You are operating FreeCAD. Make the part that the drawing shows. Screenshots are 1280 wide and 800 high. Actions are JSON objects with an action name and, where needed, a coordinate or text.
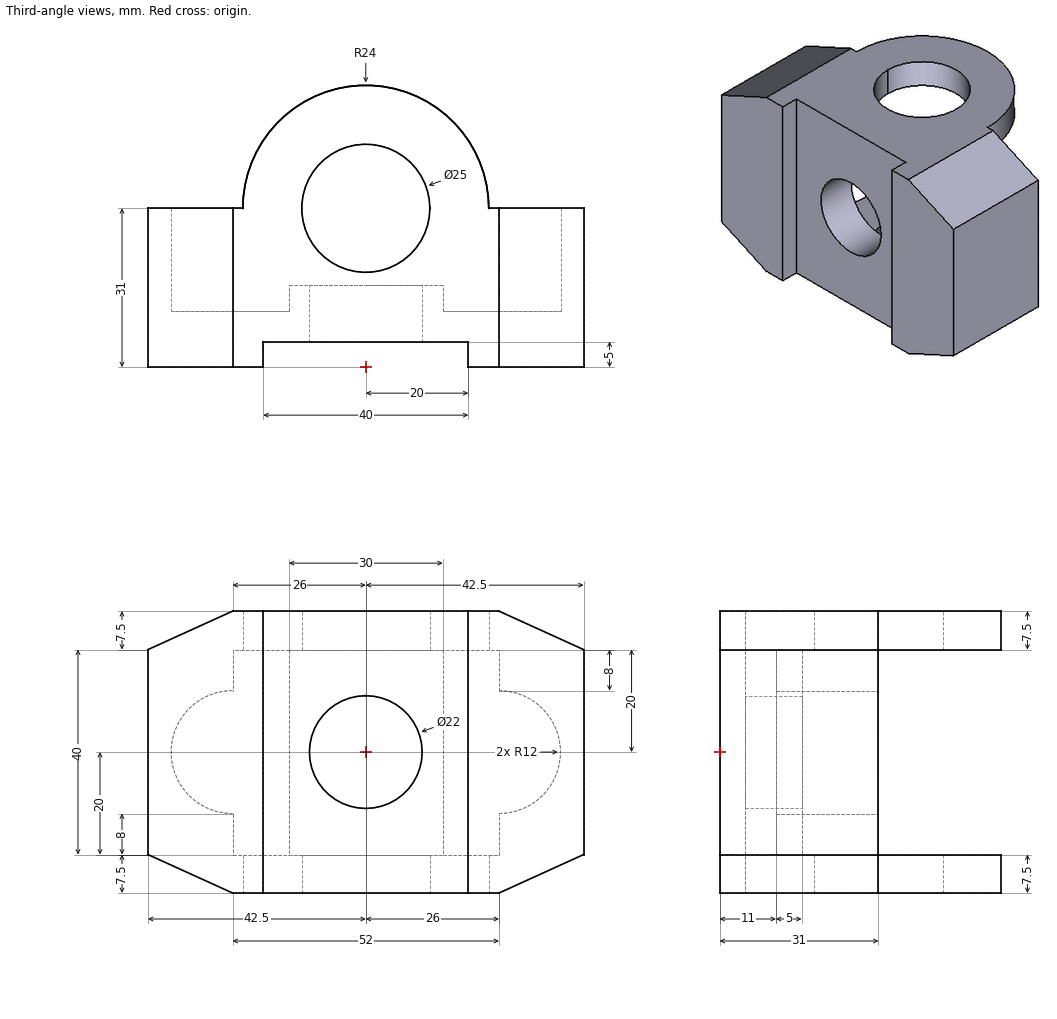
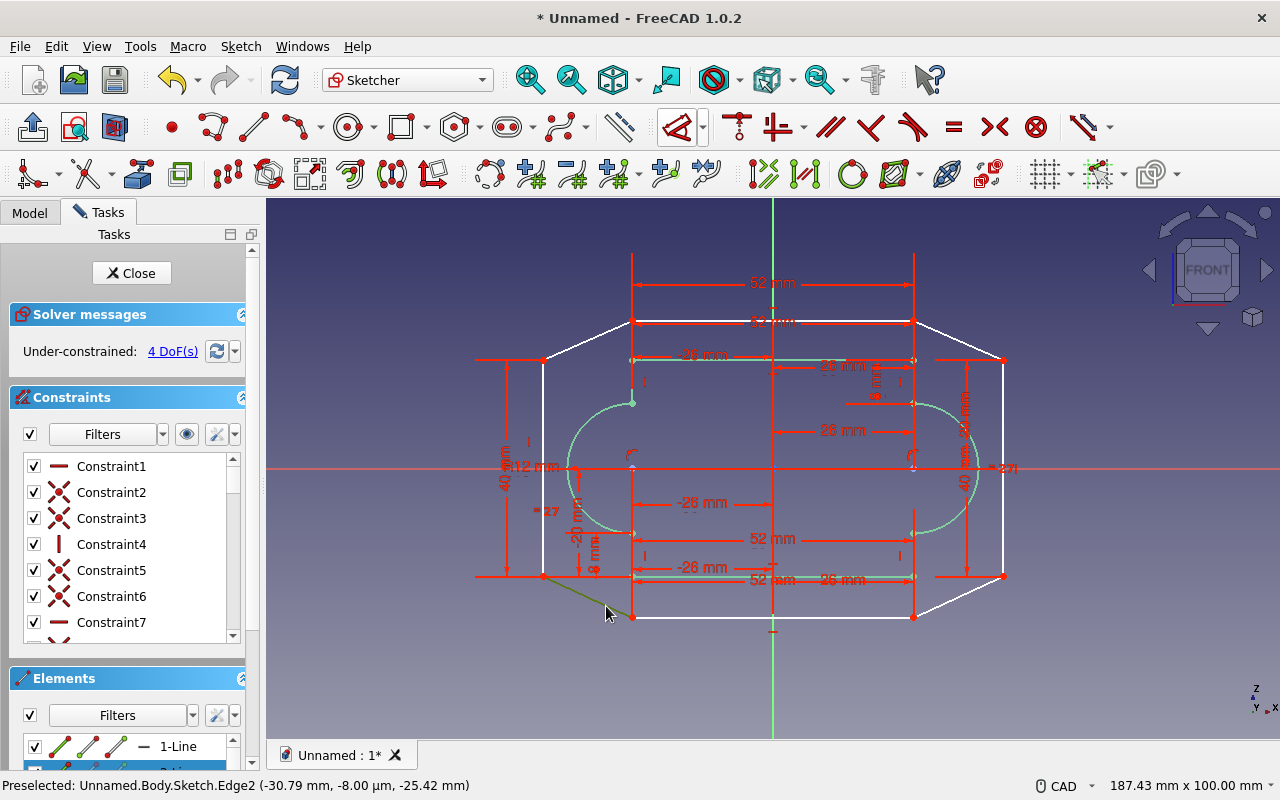
{"action": "left_click", "coordinate": [702, 128]}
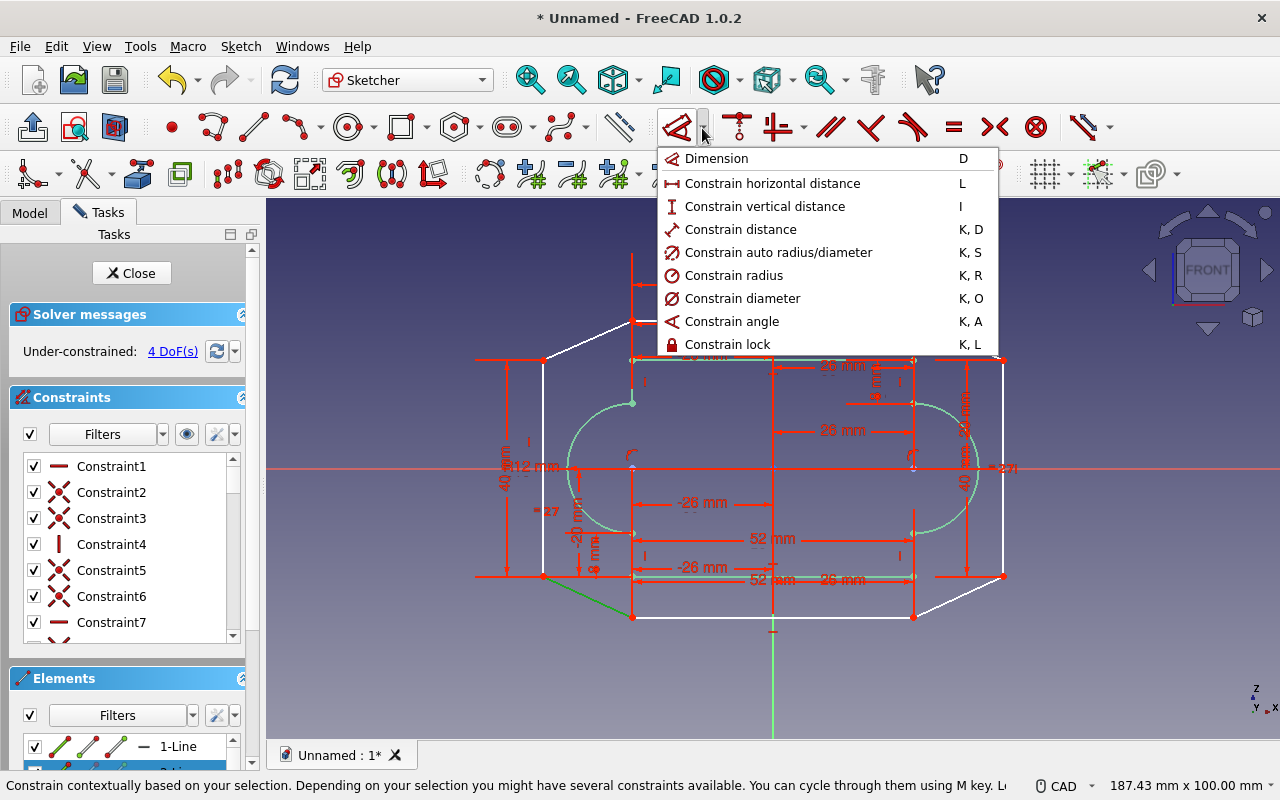
{"action": "left_click", "coordinate": [828, 206]}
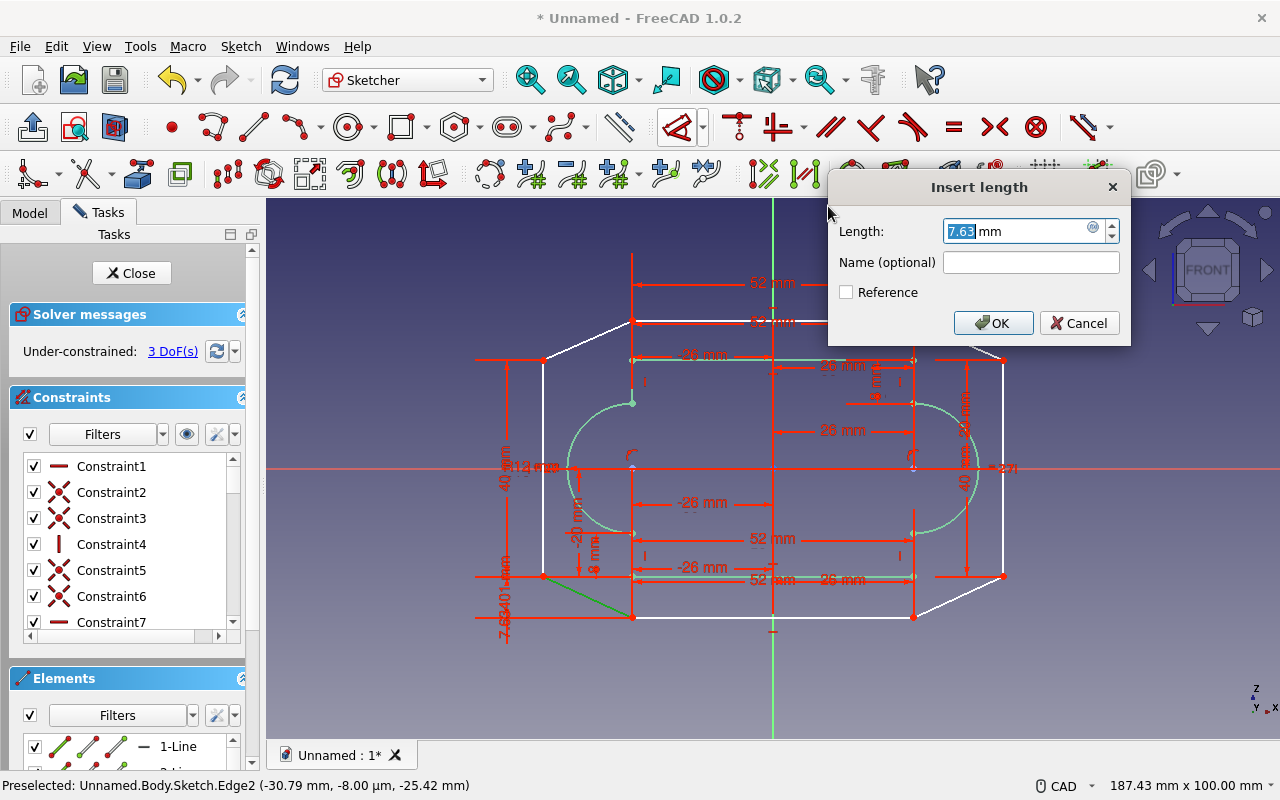
{"action": "type", "text": "7.5"}
{"action": "key", "text": "Return"}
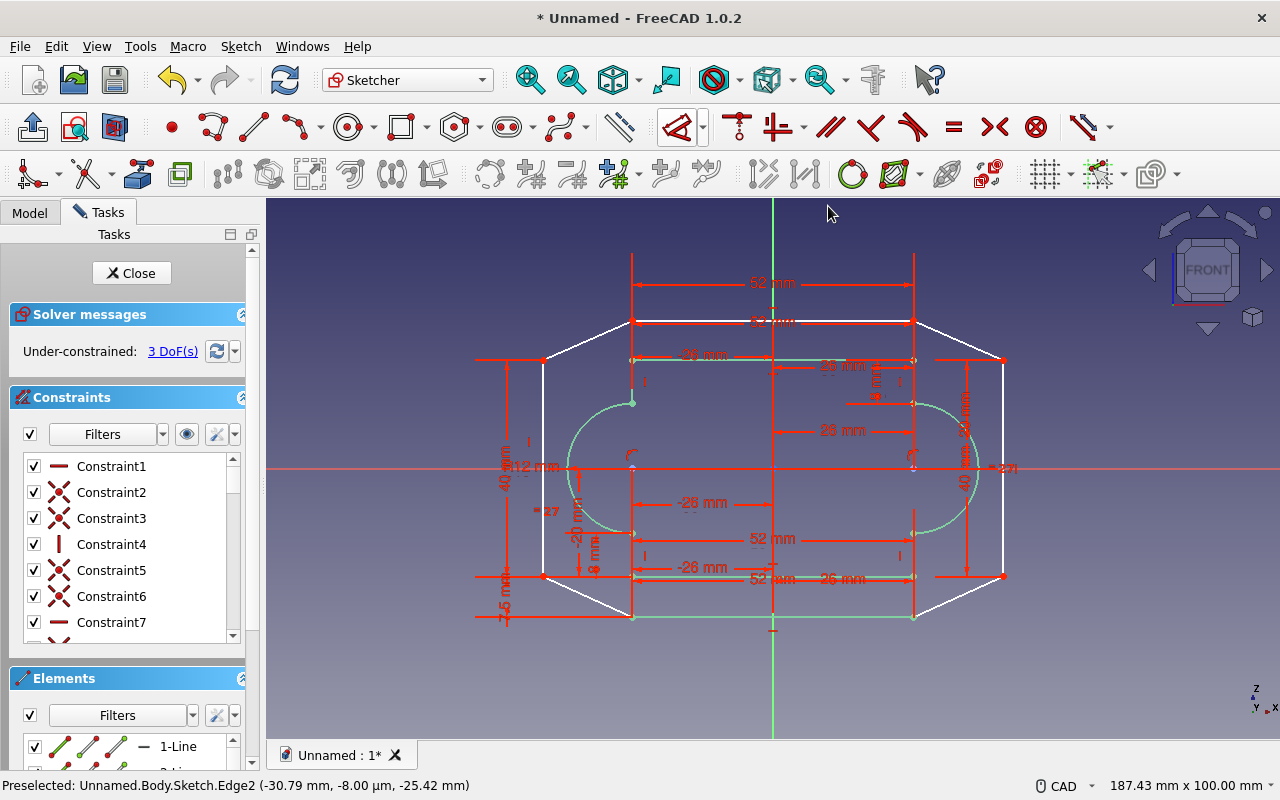
{"action": "left_click", "coordinate": [570, 349]}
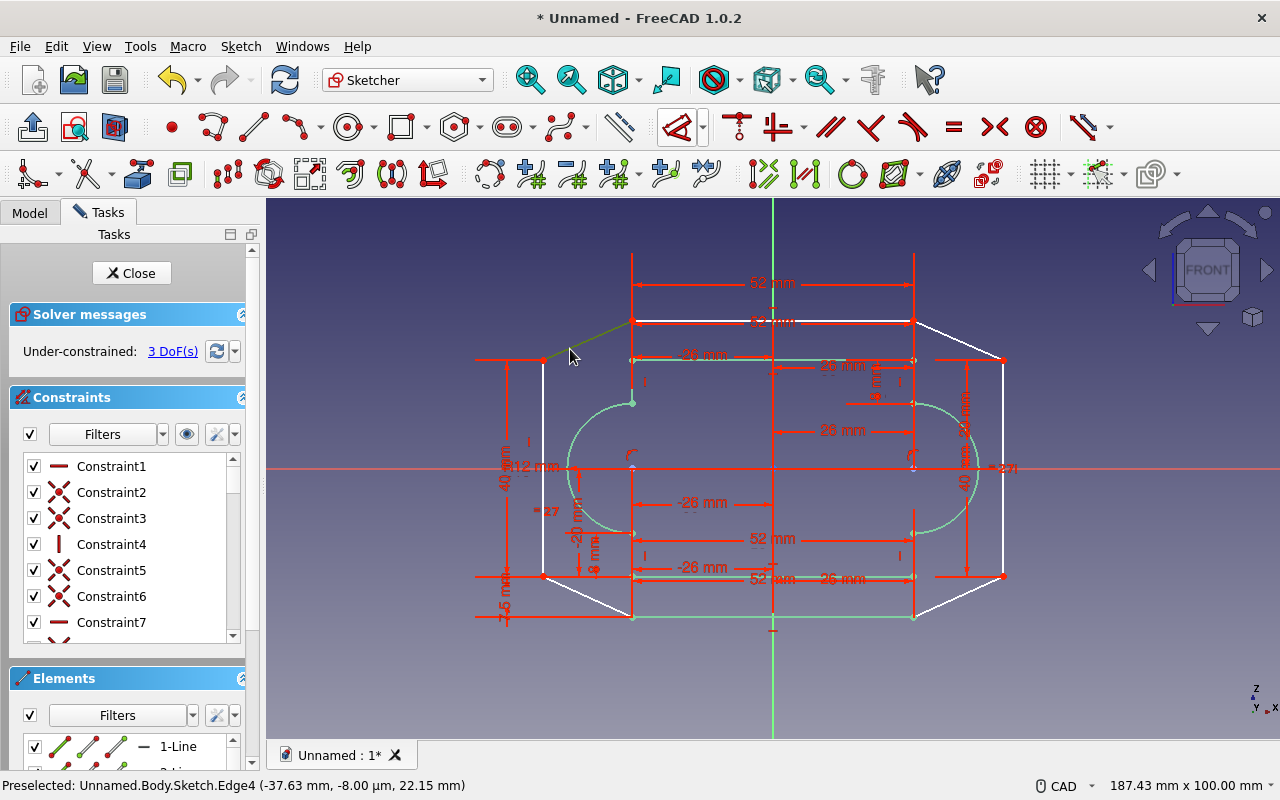
{"action": "key", "text": "i"}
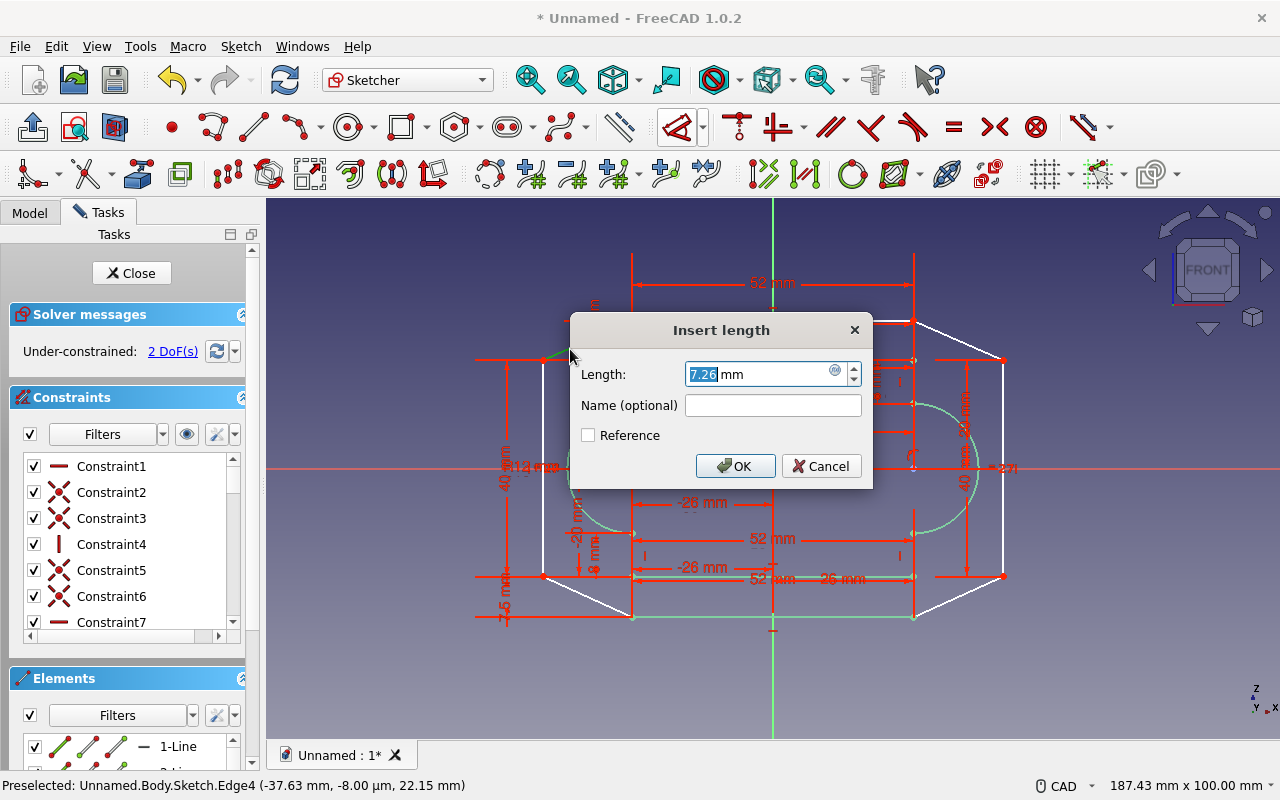
{"action": "type", "text": "7.5"}
{"action": "key", "text": "Return"}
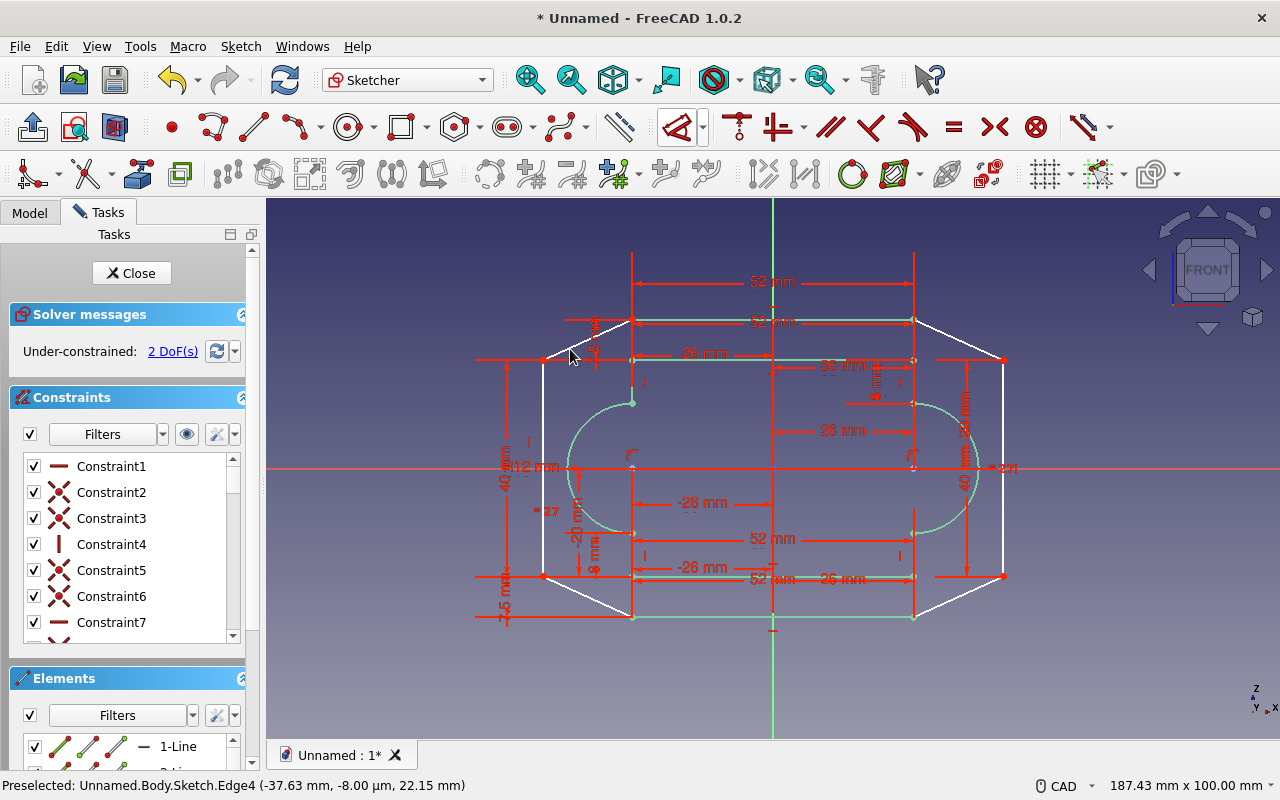
{"action": "left_click", "coordinate": [543, 577]}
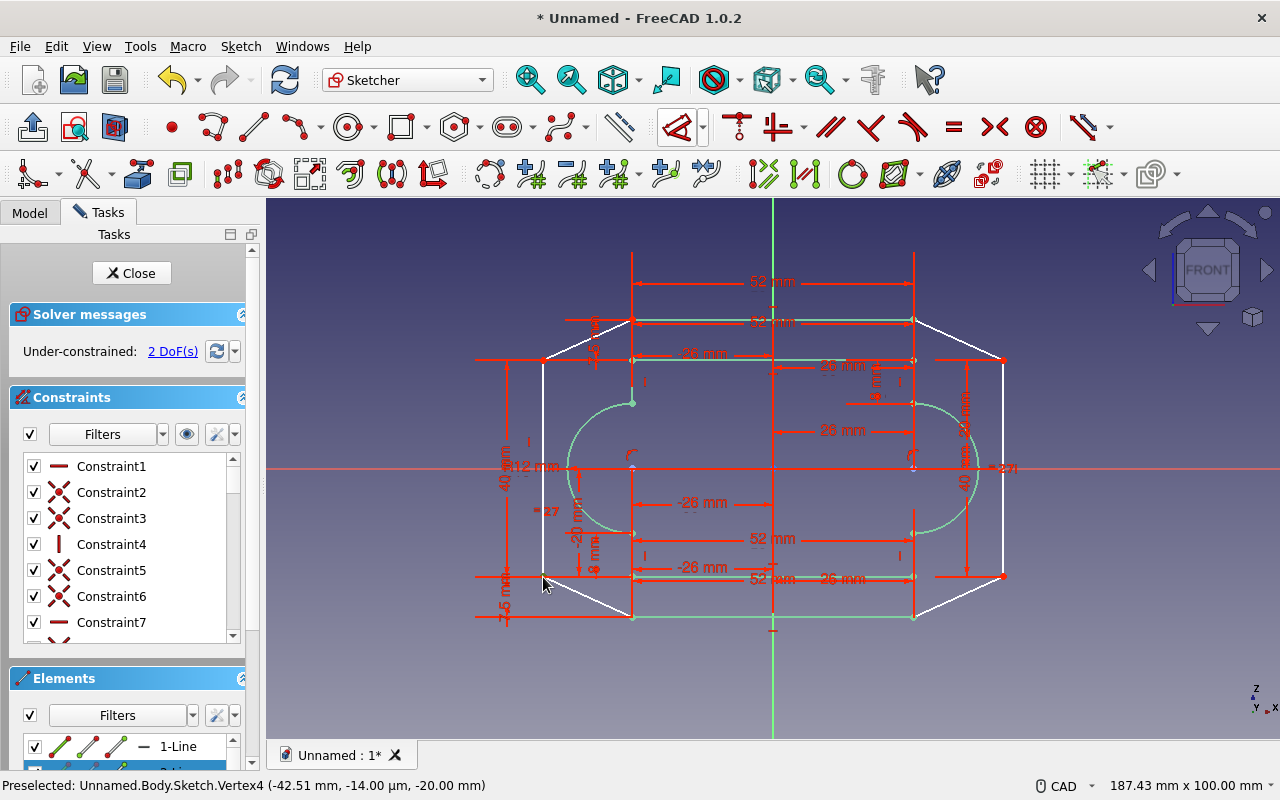
{"action": "left_click", "coordinate": [702, 128]}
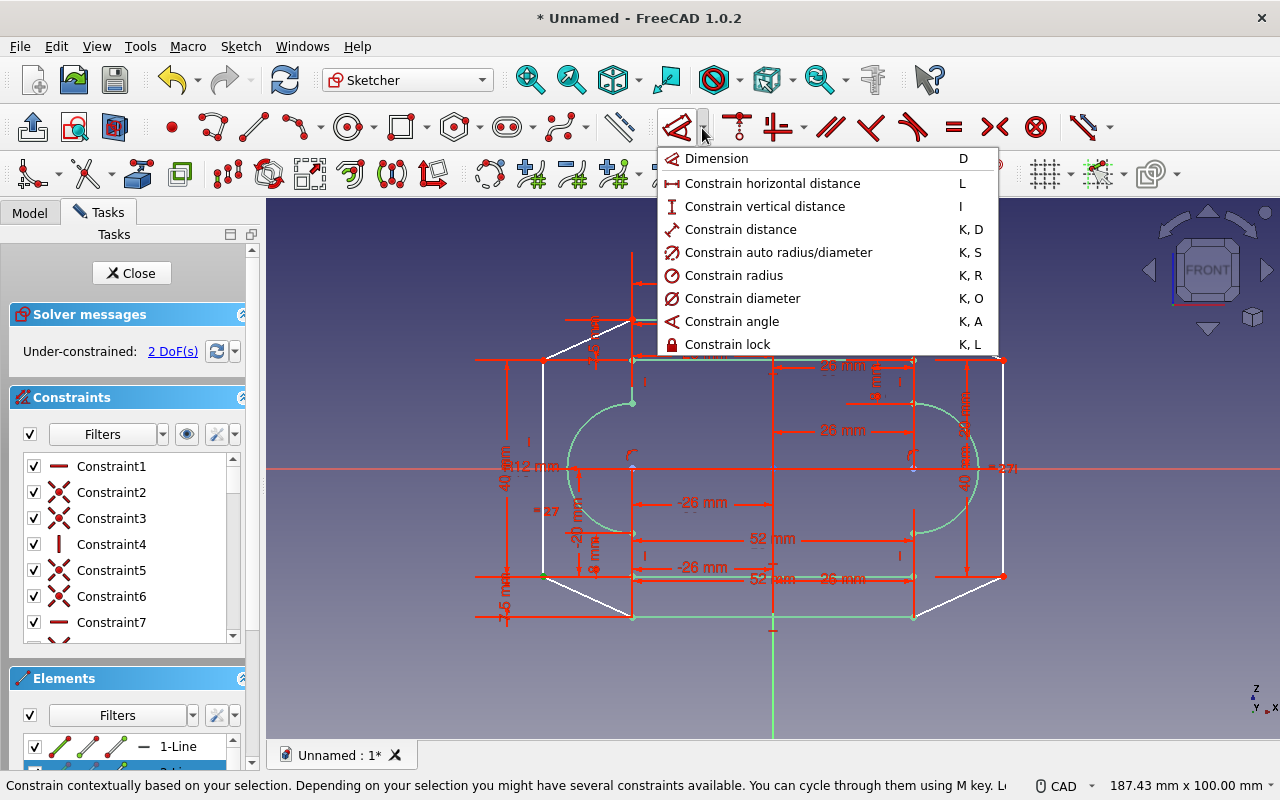
{"action": "left_click", "coordinate": [828, 184]}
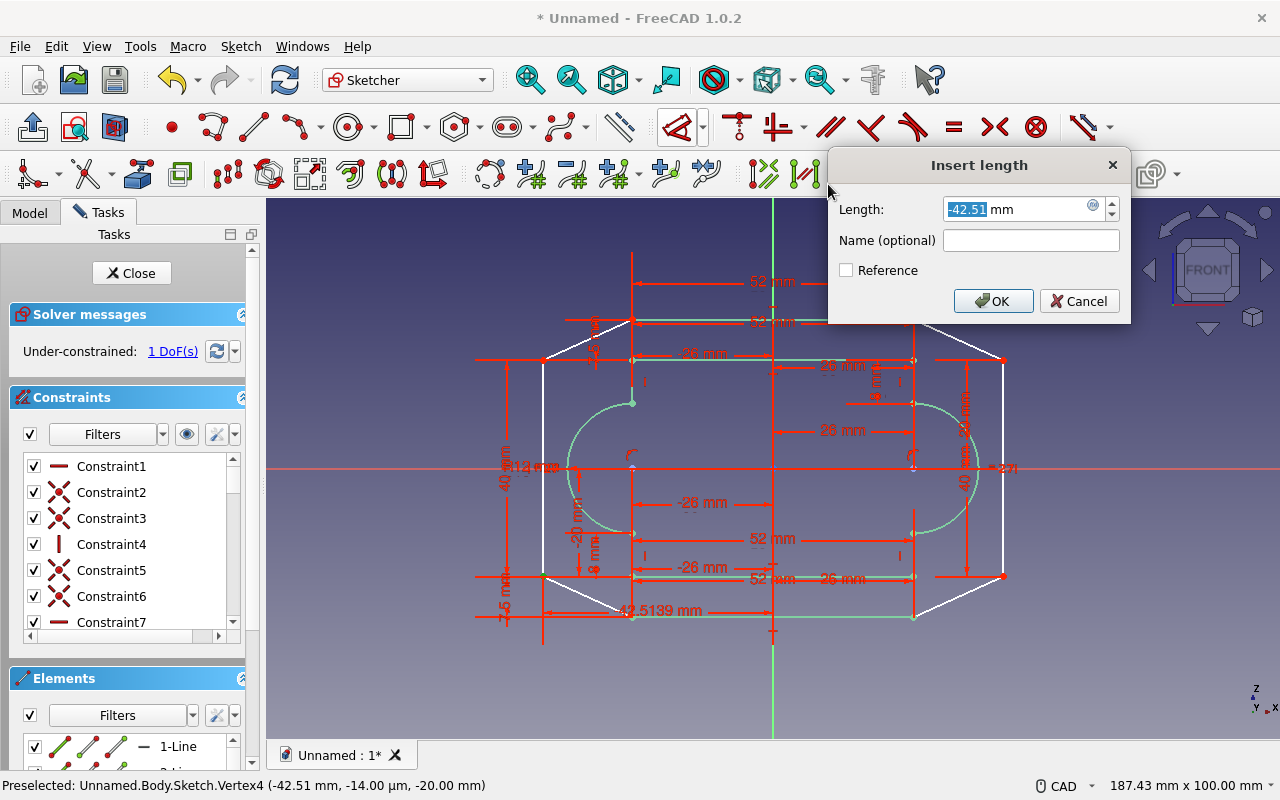
{"action": "type", "text": "-42.5"}
{"action": "key", "text": "Return"}